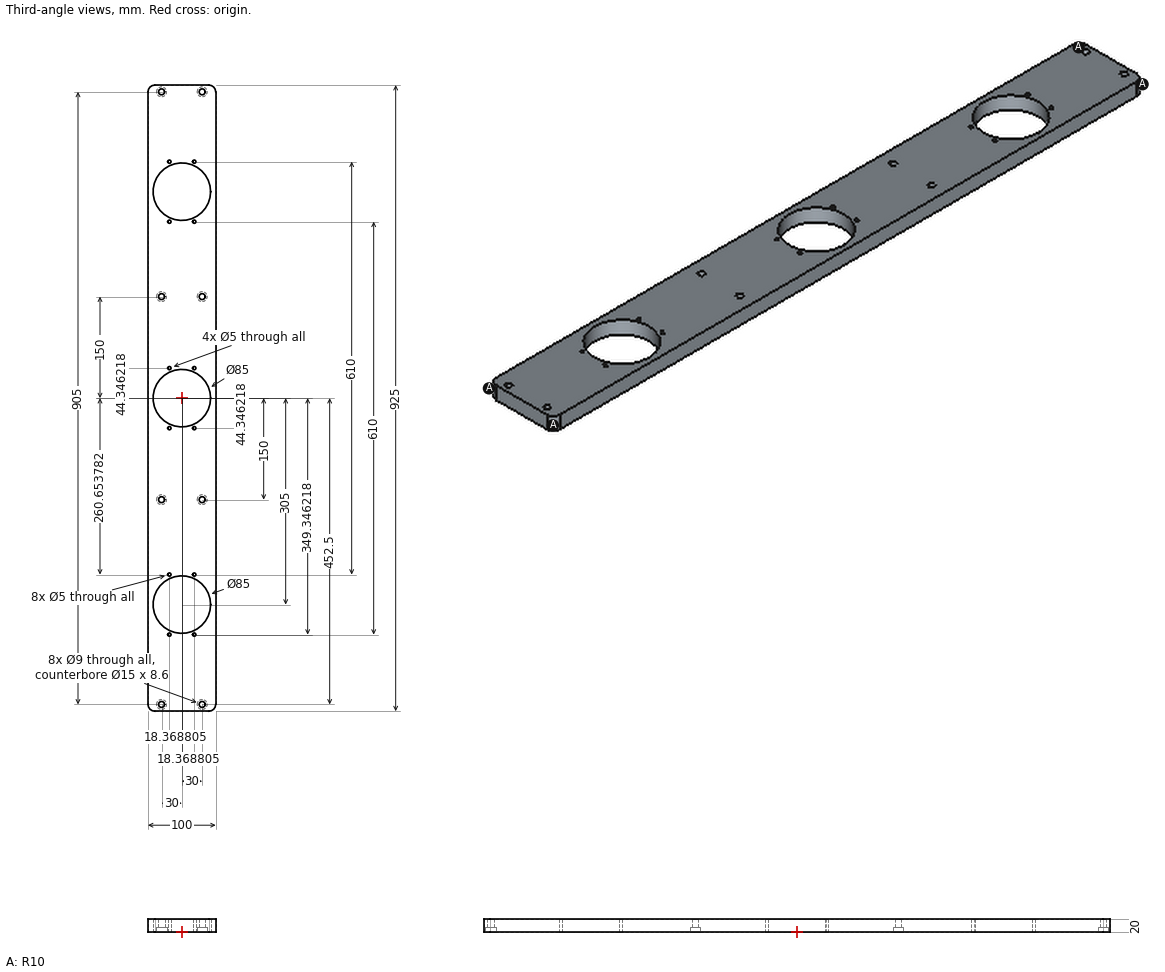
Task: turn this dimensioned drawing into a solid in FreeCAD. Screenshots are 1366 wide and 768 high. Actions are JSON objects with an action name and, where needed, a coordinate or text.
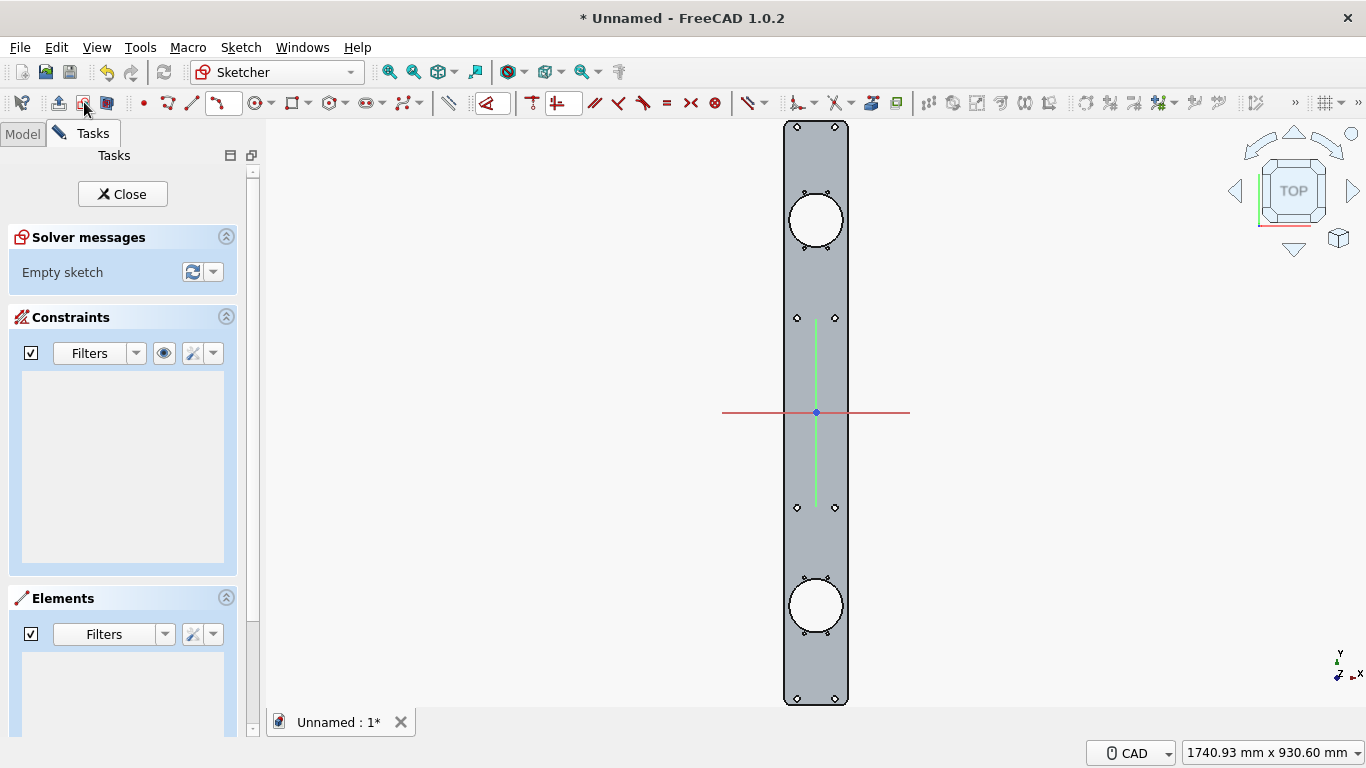
{"action": "scroll", "coordinate": [827, 413], "scroll_direction": "up", "scroll_amount": 10}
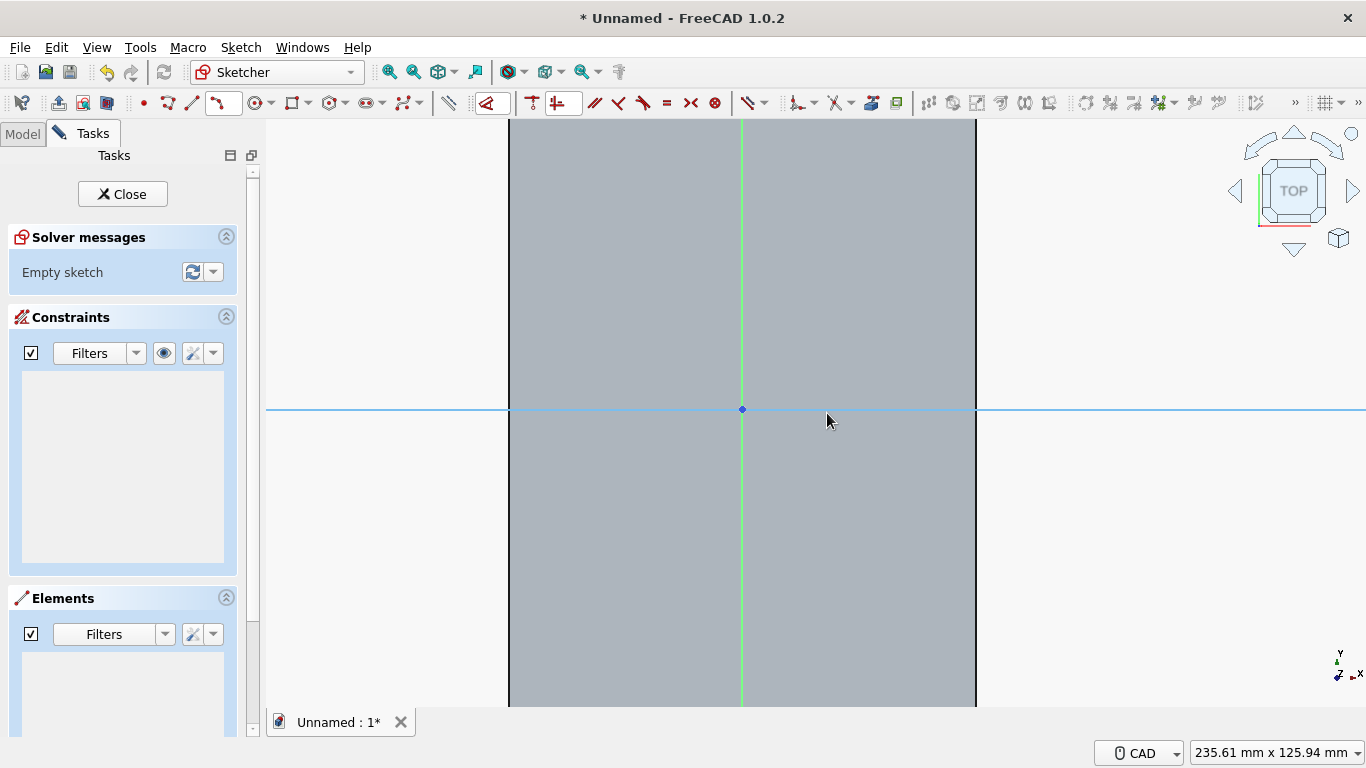
{"action": "key", "text": "g c"}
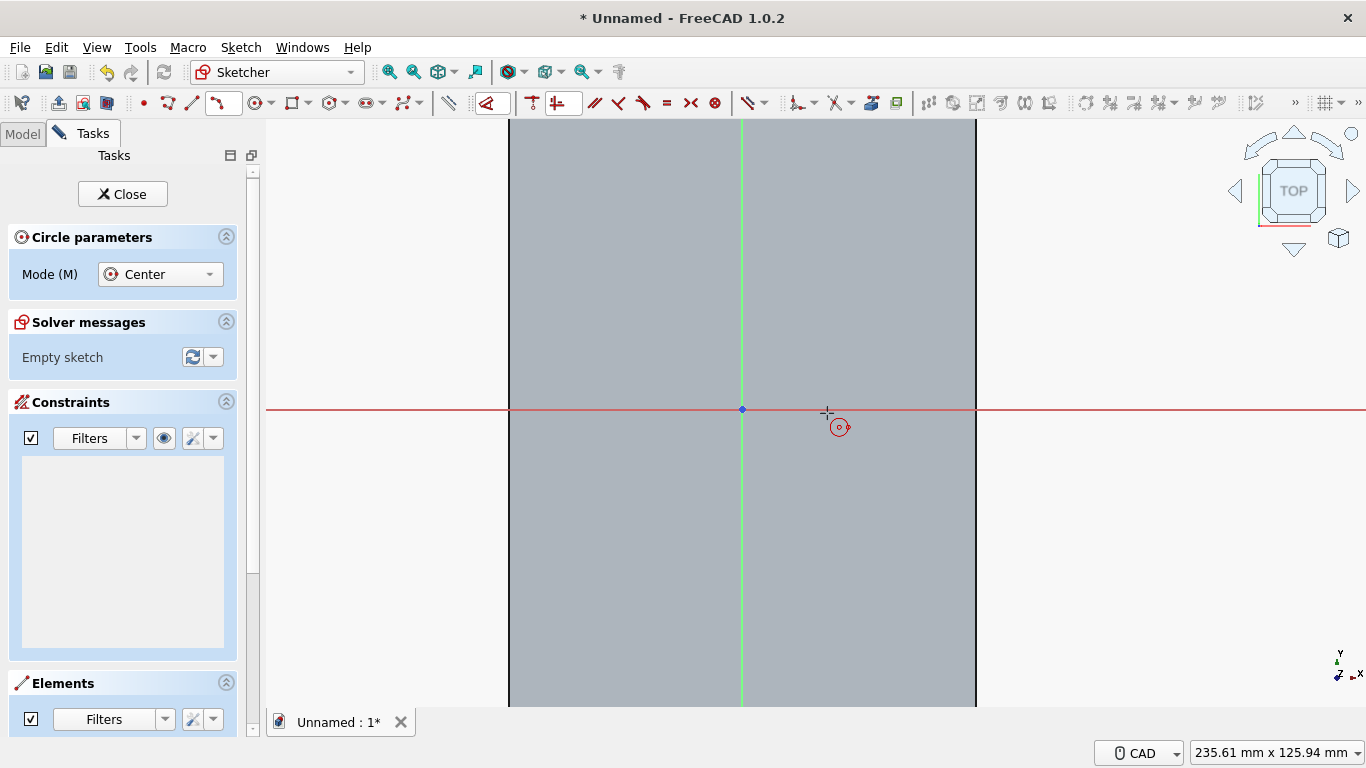
{"action": "left_click", "coordinate": [742, 410]}
{"action": "left_click", "coordinate": [883, 269]}
{"action": "key", "text": "Escape"}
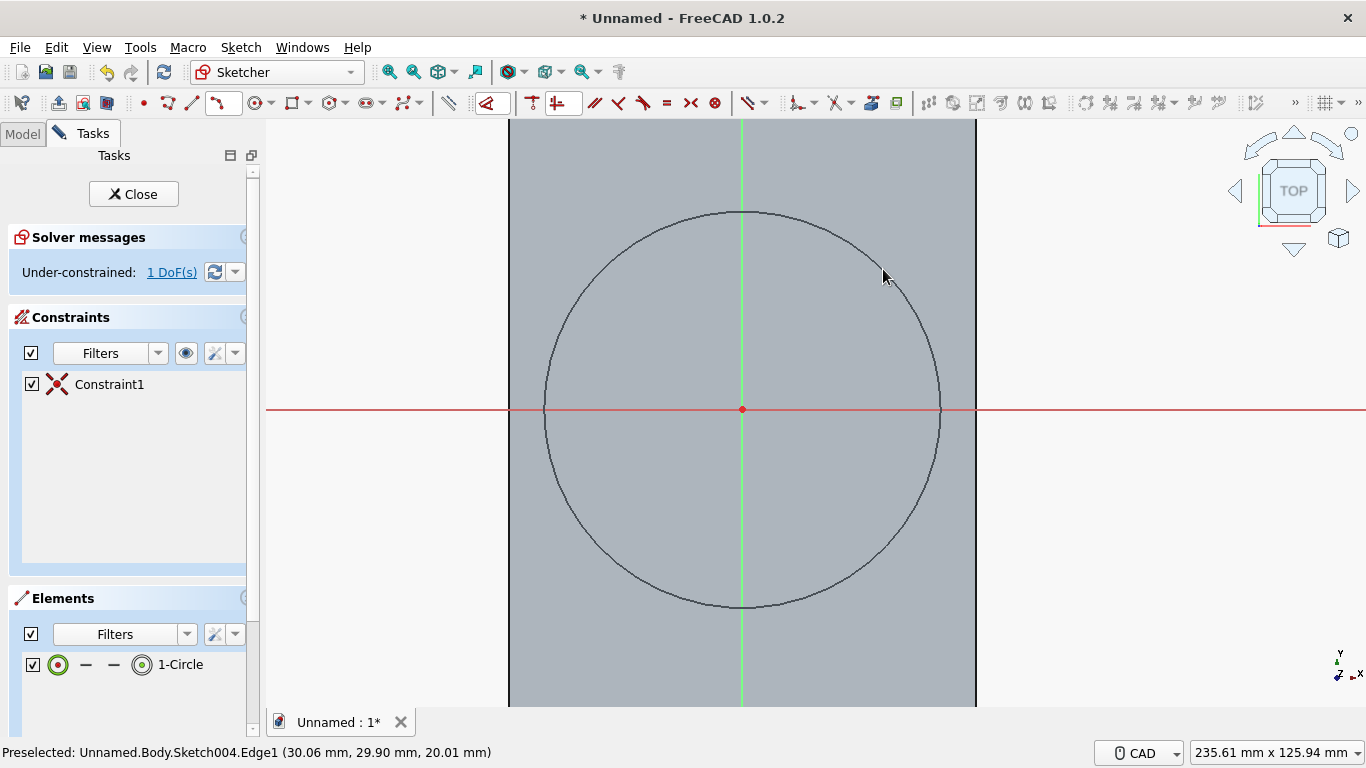
{"action": "left_click", "coordinate": [486, 104]}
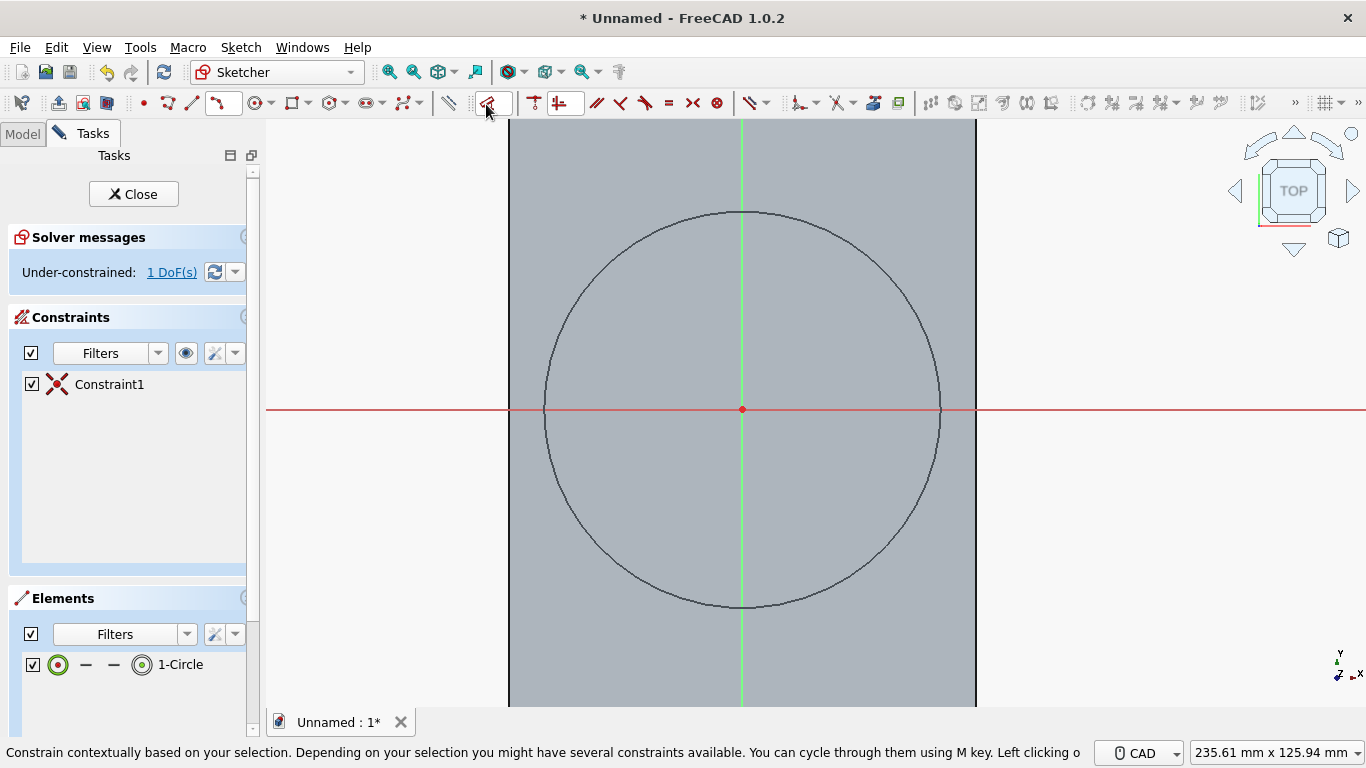
{"action": "left_click", "coordinate": [882, 269]}
{"action": "left_click", "coordinate": [905, 246]}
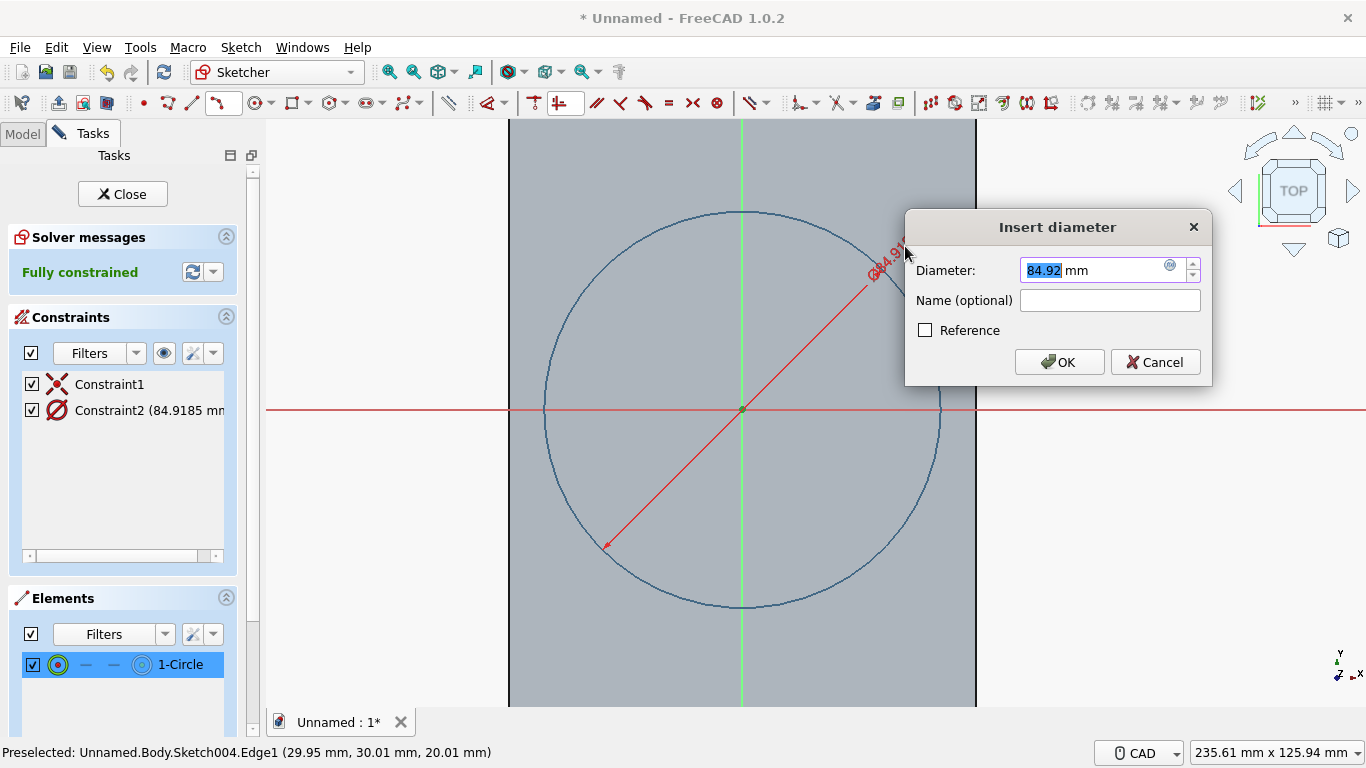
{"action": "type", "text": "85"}
{"action": "key", "text": "Return"}
{"action": "key", "text": "Escape"}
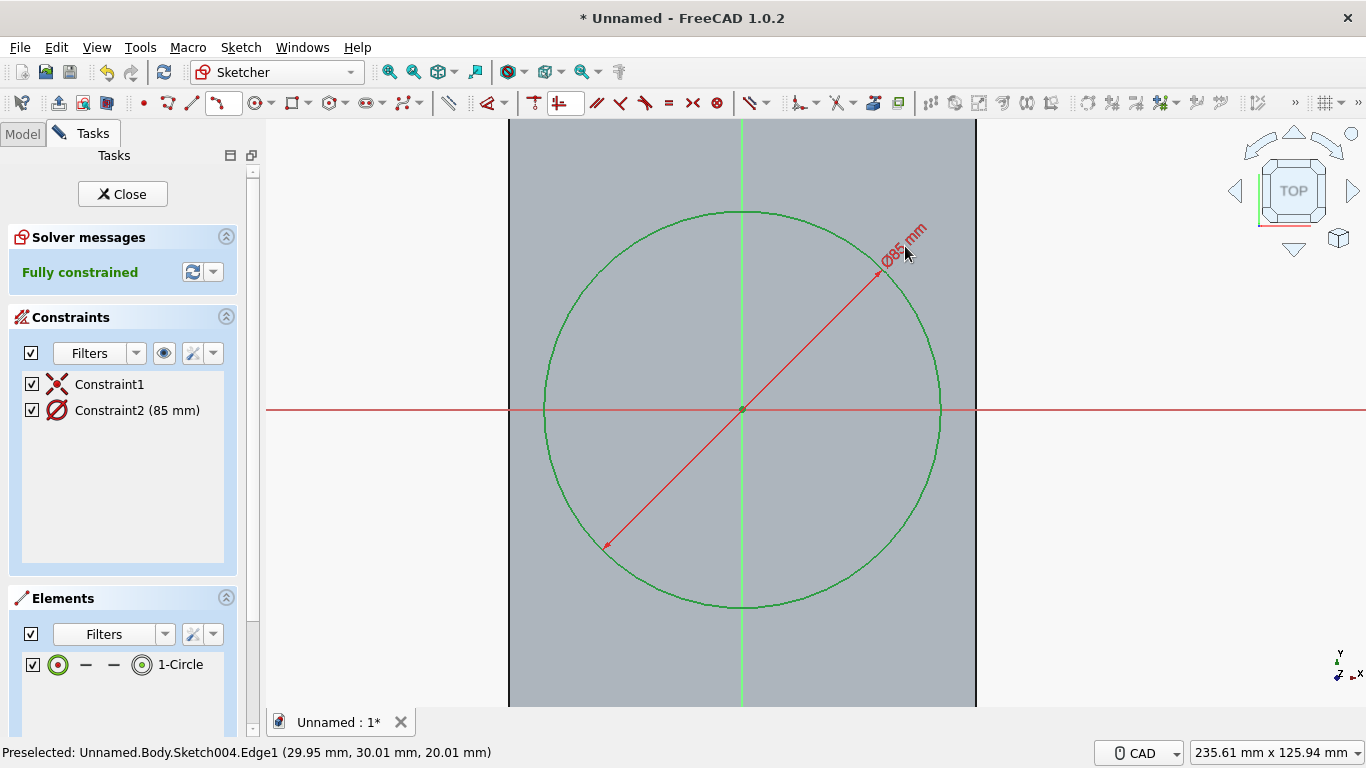
{"action": "left_click", "coordinate": [123, 194]}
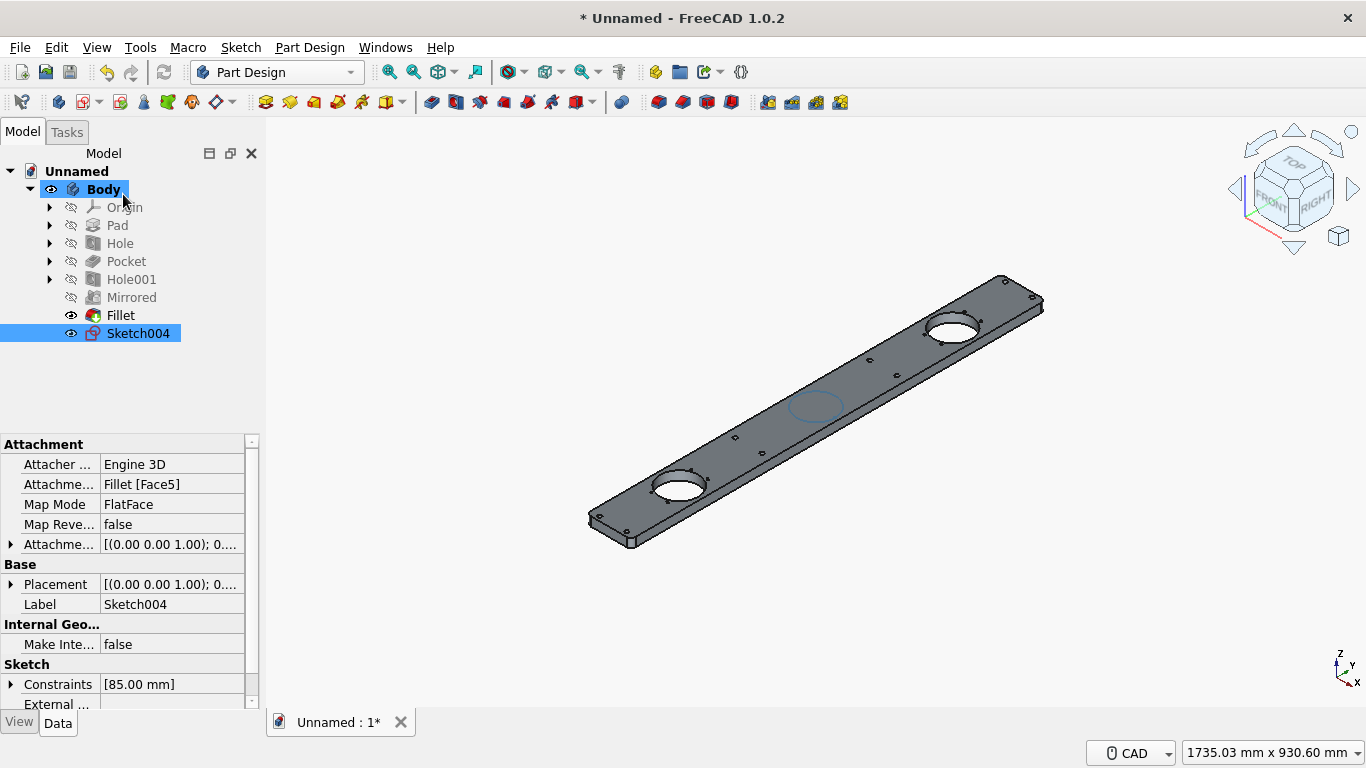
{"action": "left_click", "coordinate": [432, 102]}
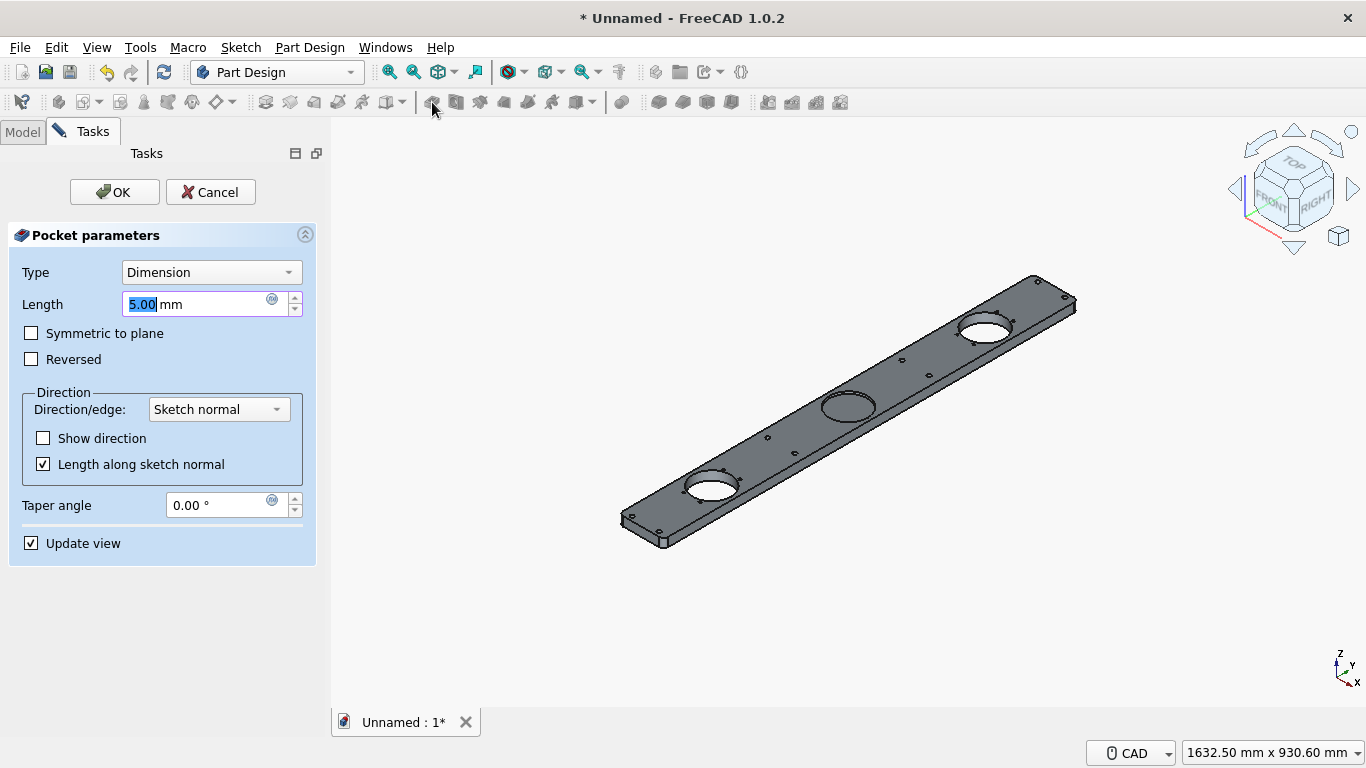
{"action": "left_click", "coordinate": [212, 272]}